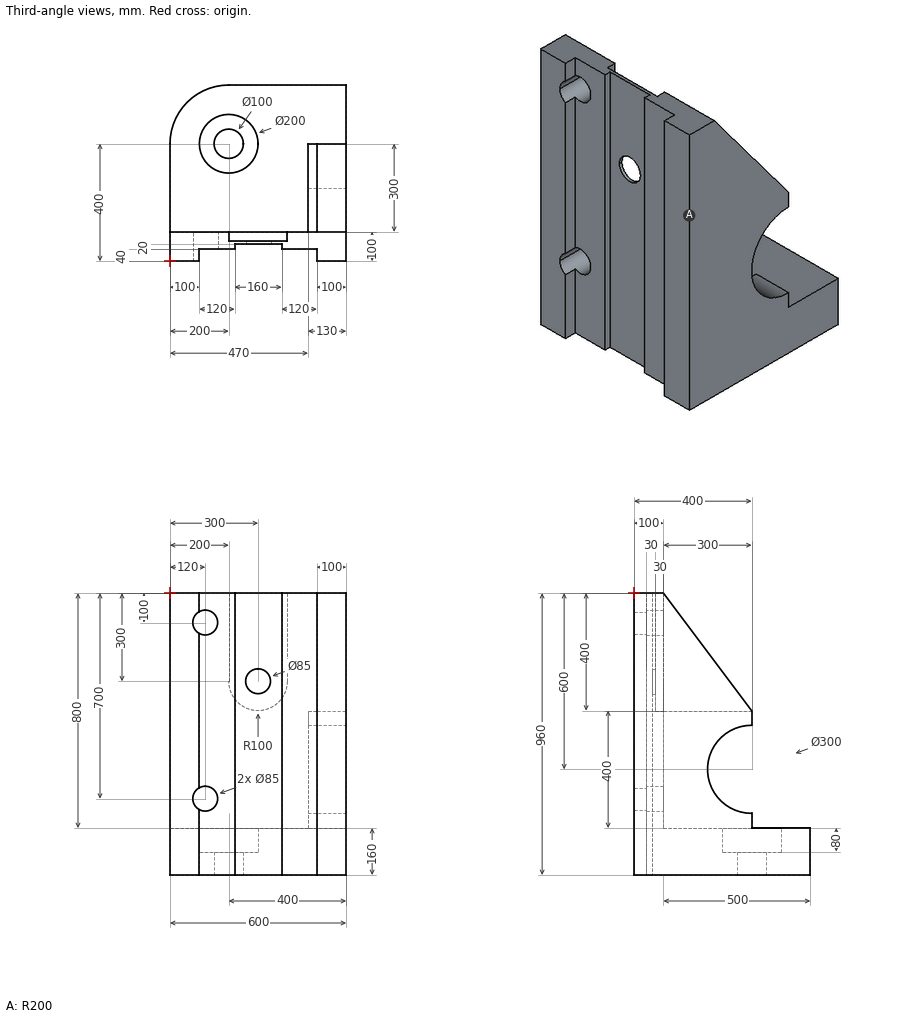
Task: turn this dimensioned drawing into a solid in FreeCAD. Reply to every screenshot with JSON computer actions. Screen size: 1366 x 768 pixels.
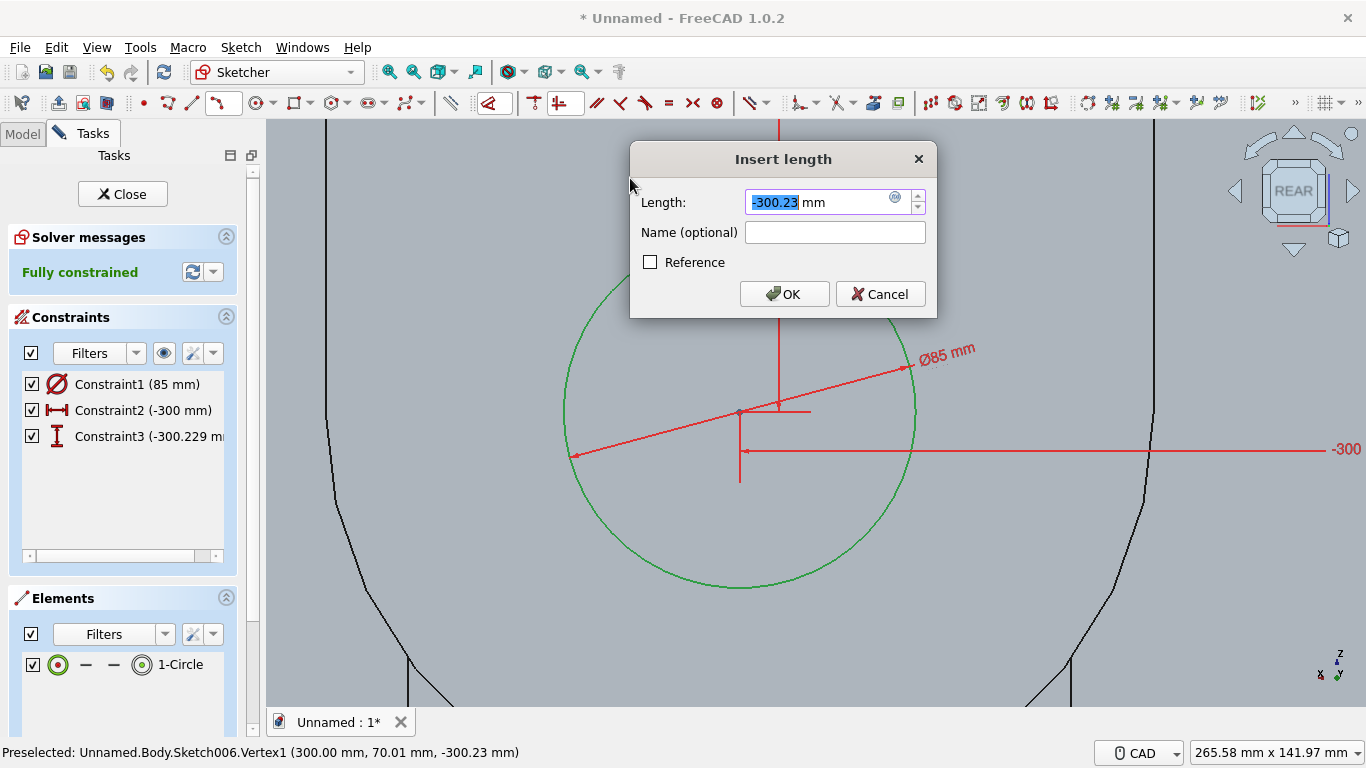
{"action": "type", "text": "-300"}
{"action": "key", "text": "Return"}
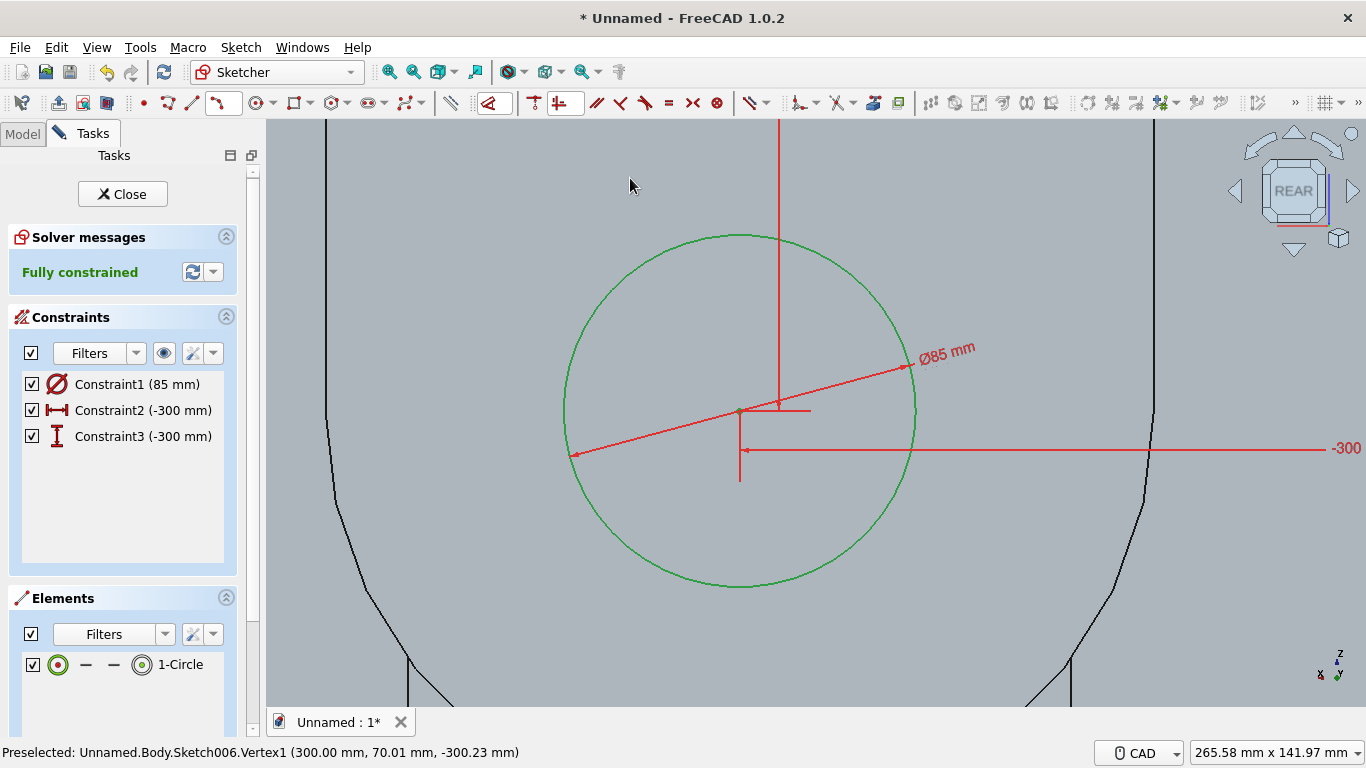
{"action": "left_click", "coordinate": [123, 194]}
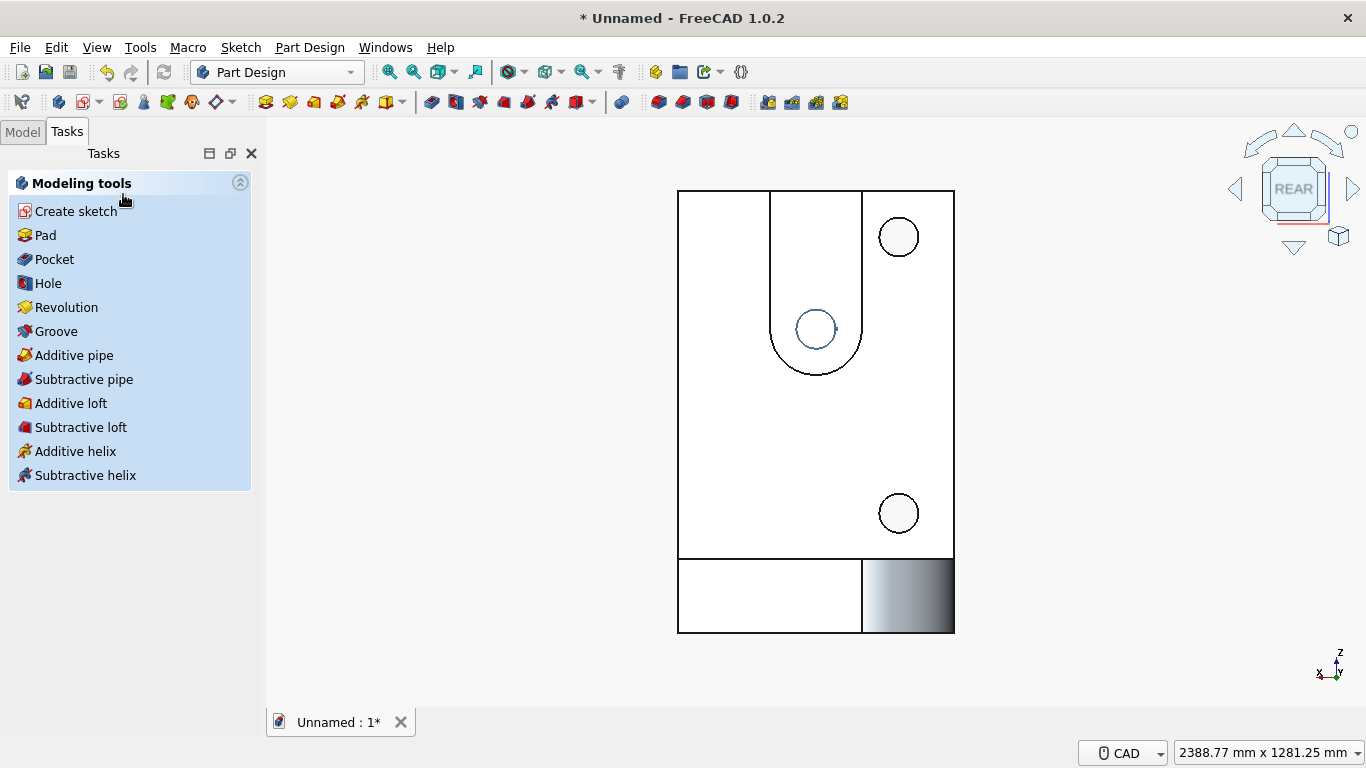
{"action": "left_click", "coordinate": [432, 102]}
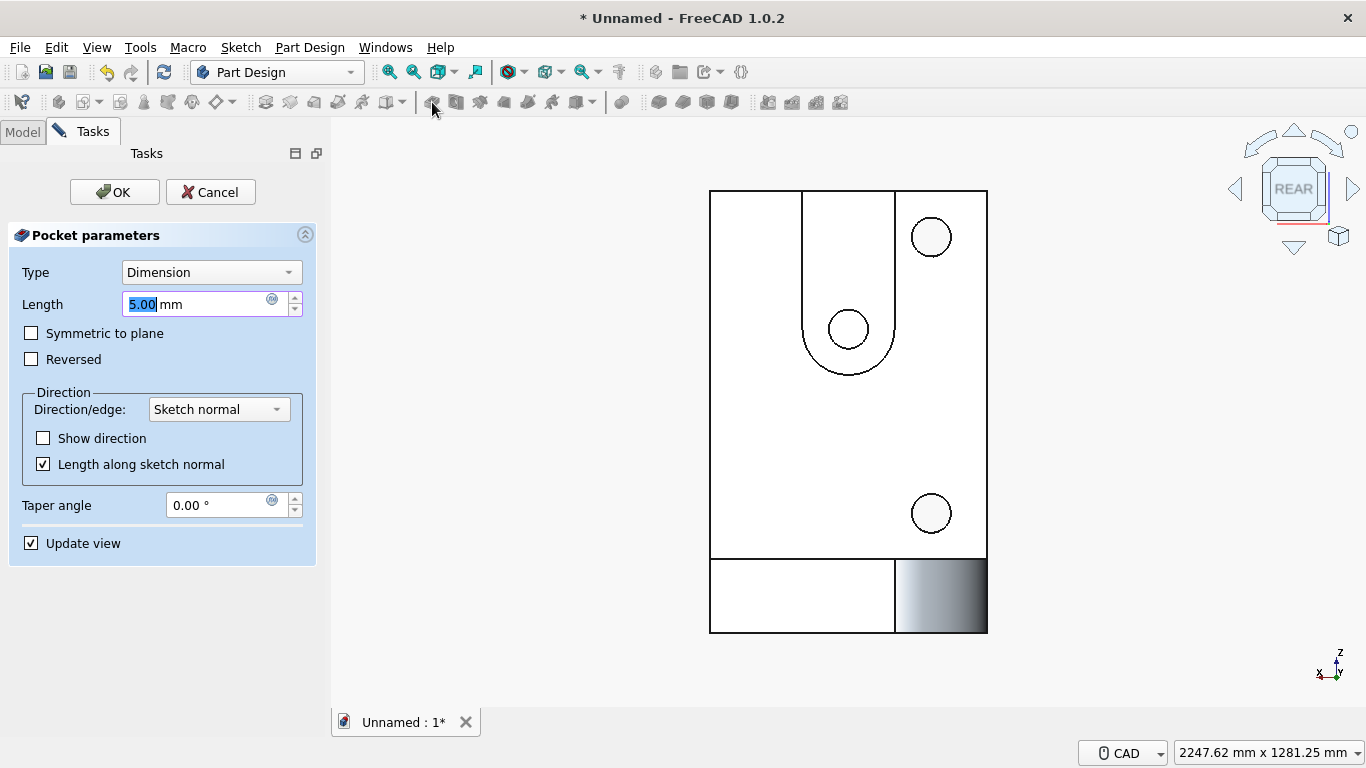
{"action": "type", "text": "30"}
{"action": "key", "text": "Tab"}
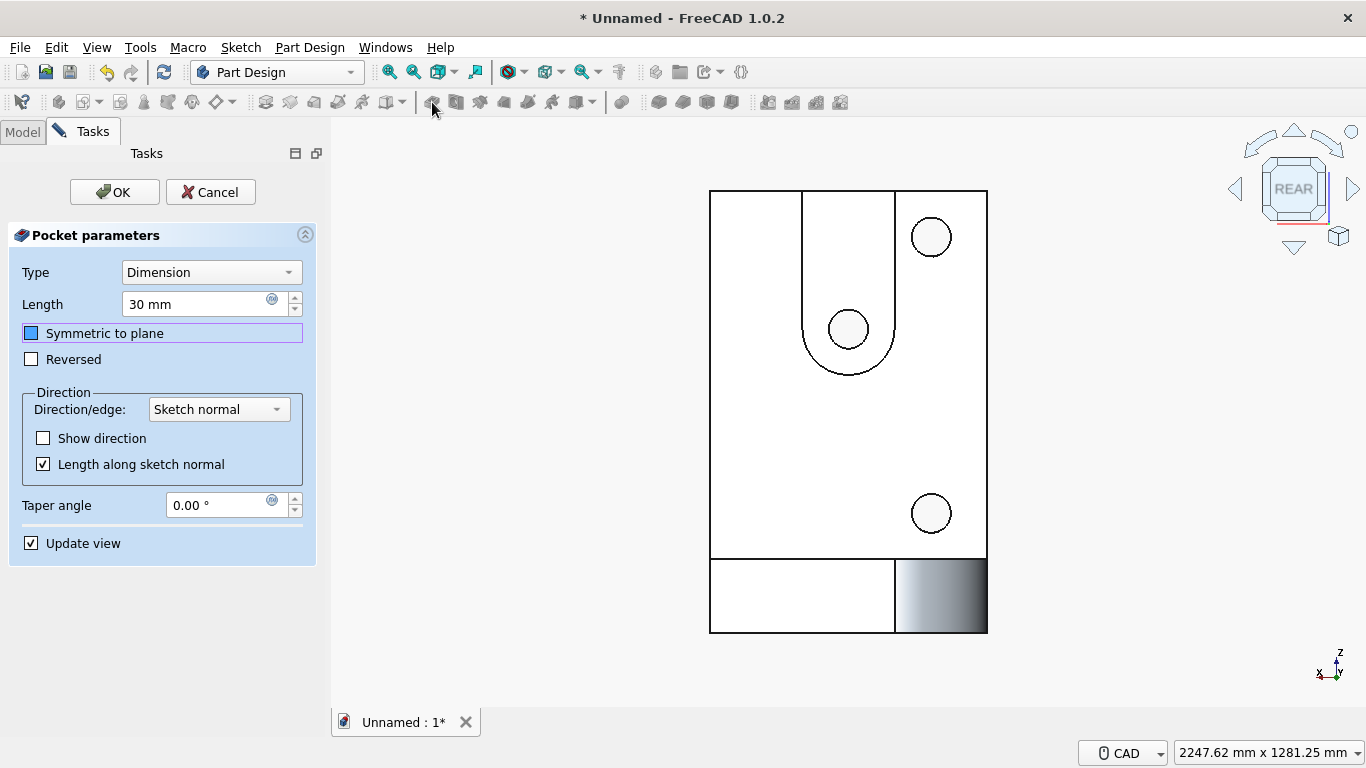
{"action": "left_click", "coordinate": [115, 192]}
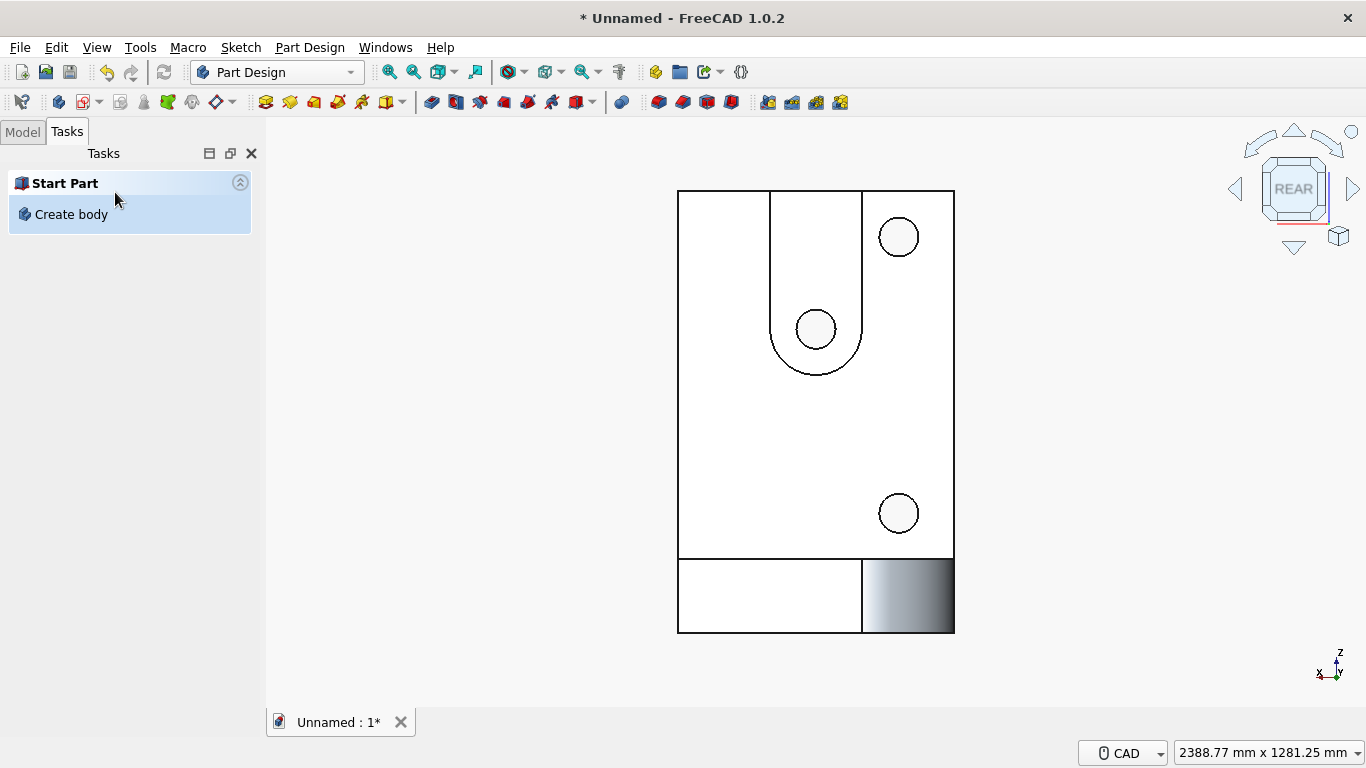
{"action": "key", "text": "0"}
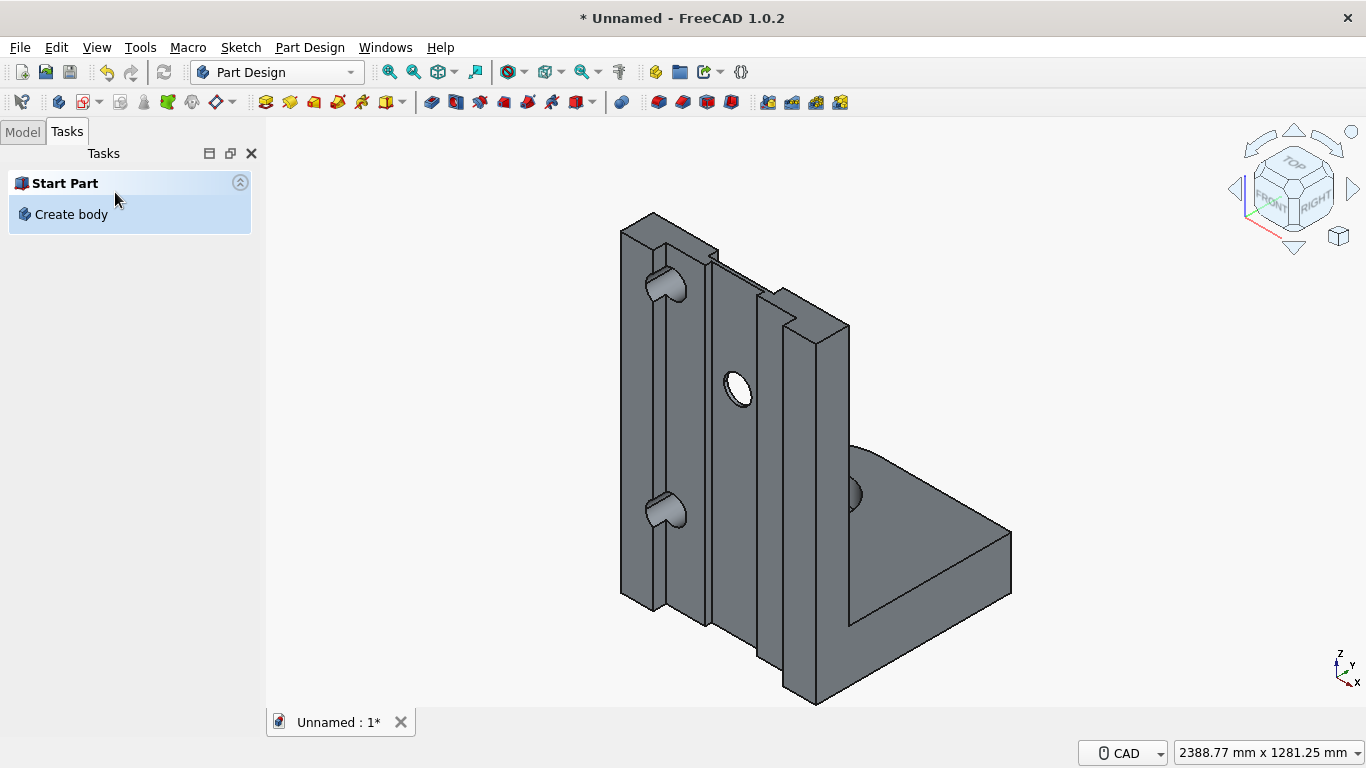
{"action": "left_click", "coordinate": [911, 541]}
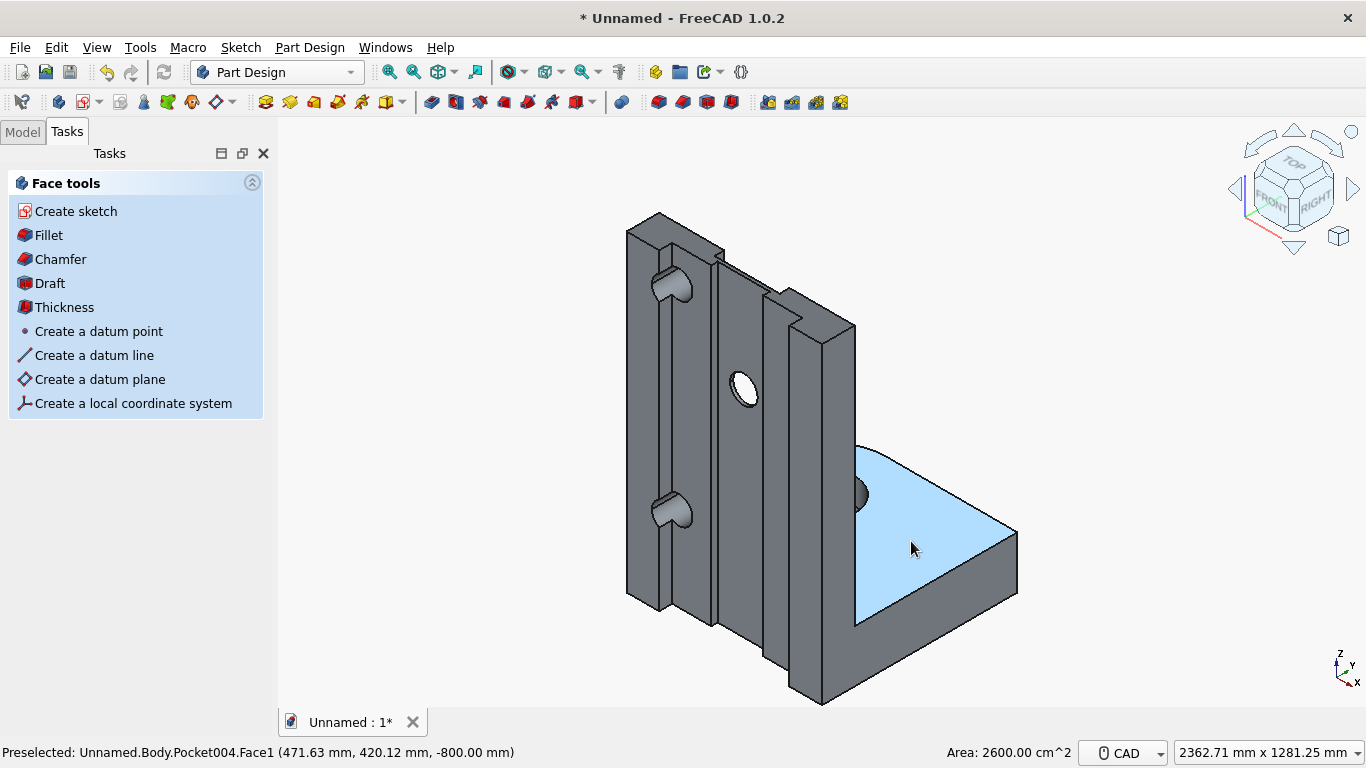
{"action": "left_click", "coordinate": [84, 102]}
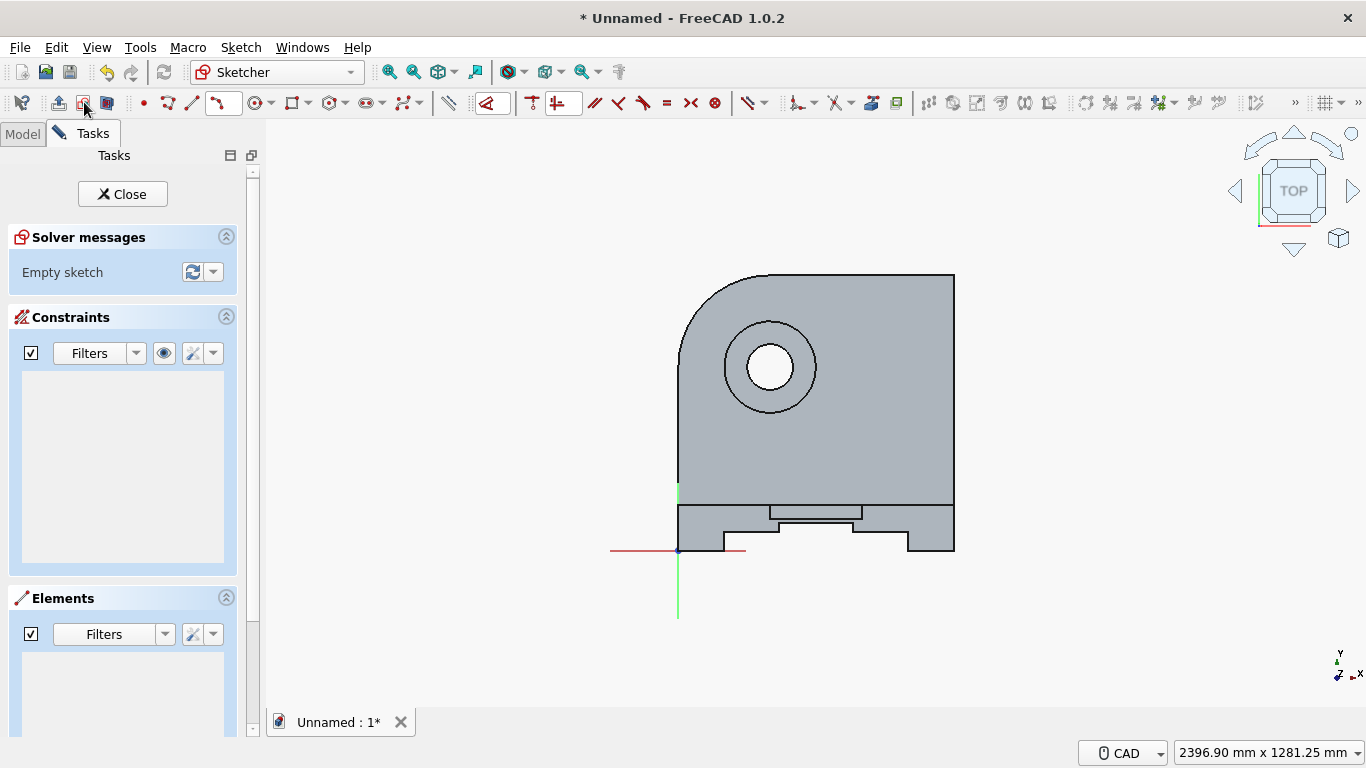
{"action": "scroll", "coordinate": [872, 496], "scroll_direction": "up", "scroll_amount": 4}